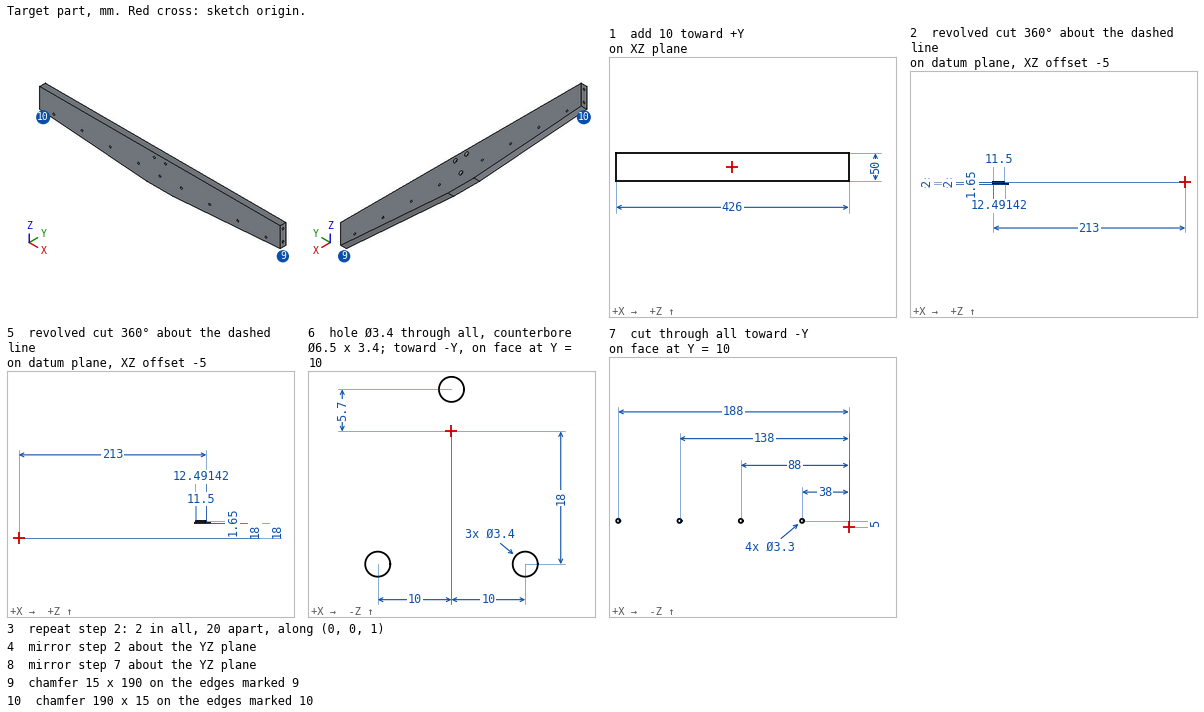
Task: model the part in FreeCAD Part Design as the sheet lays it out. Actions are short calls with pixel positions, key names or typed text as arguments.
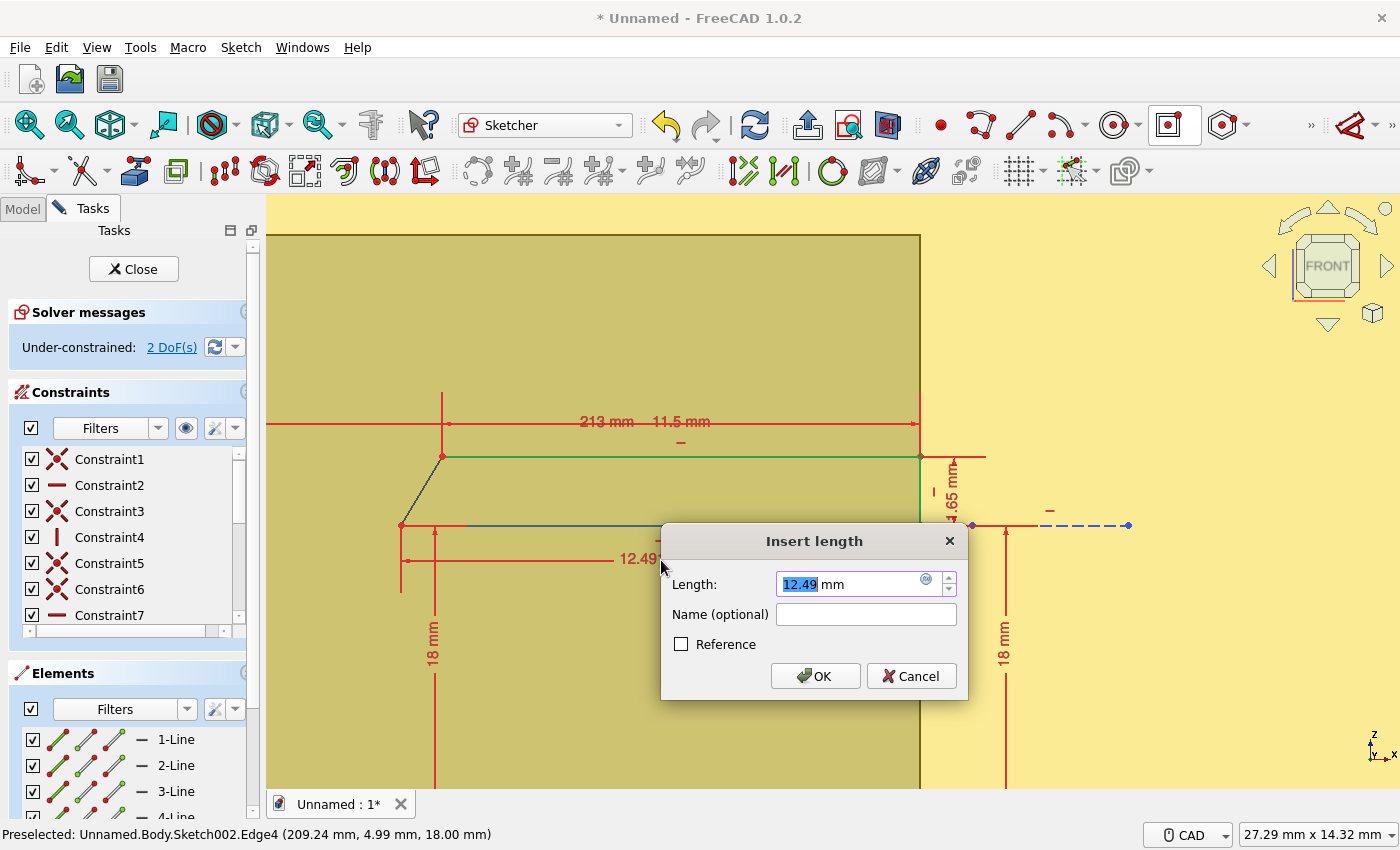
text(12.49142)
key(Return)
key(Escape)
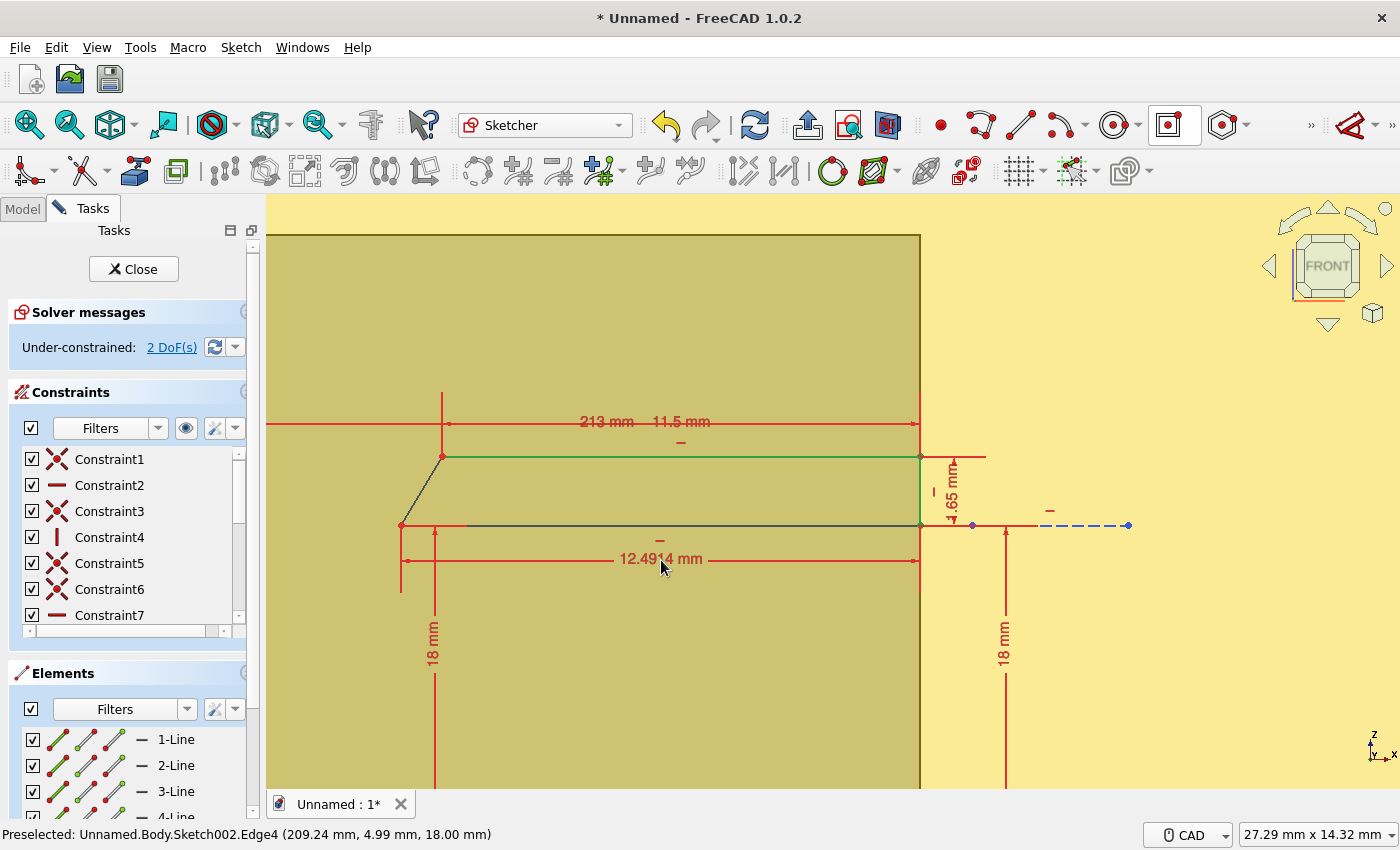
click(134, 269)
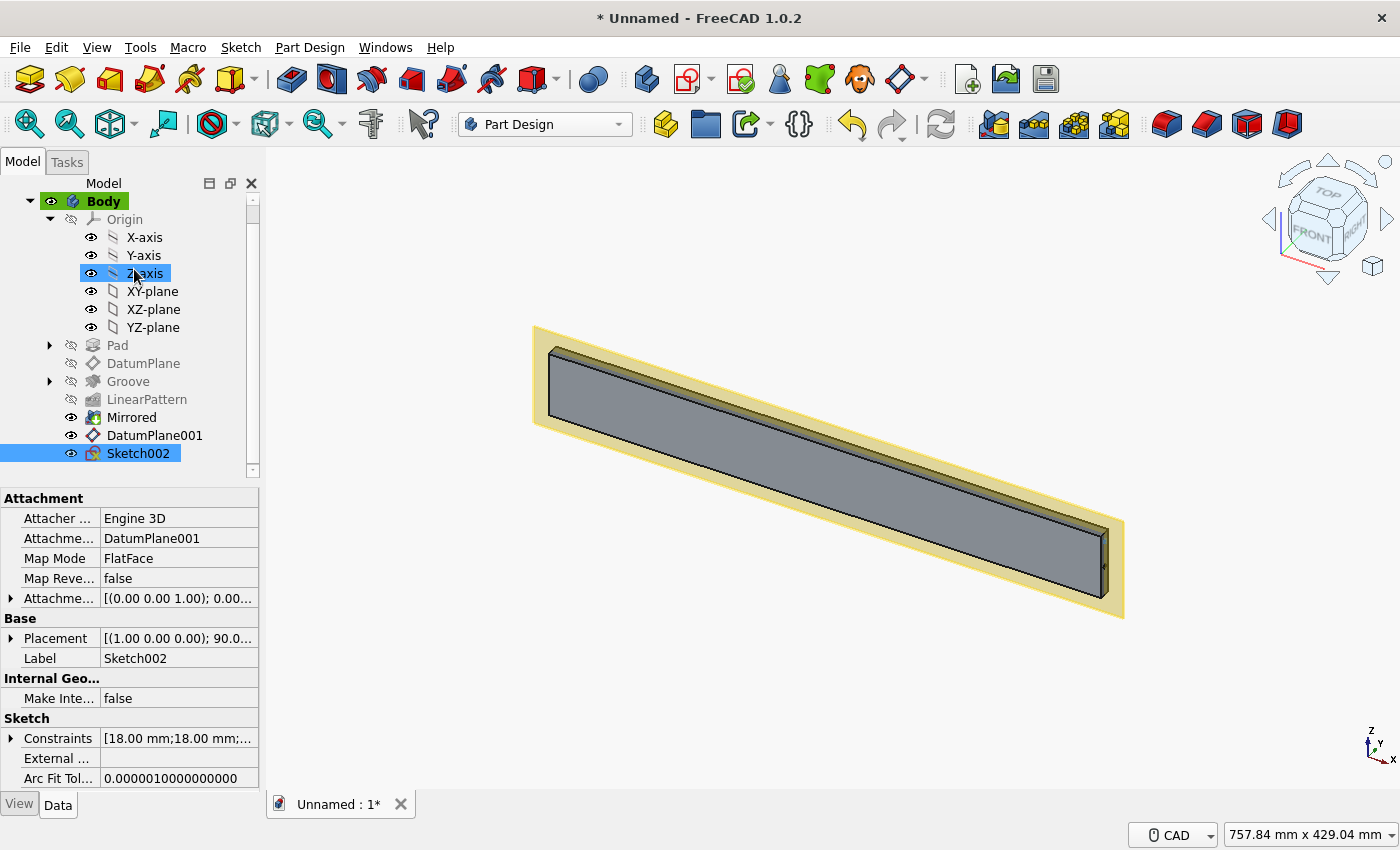
click(372, 80)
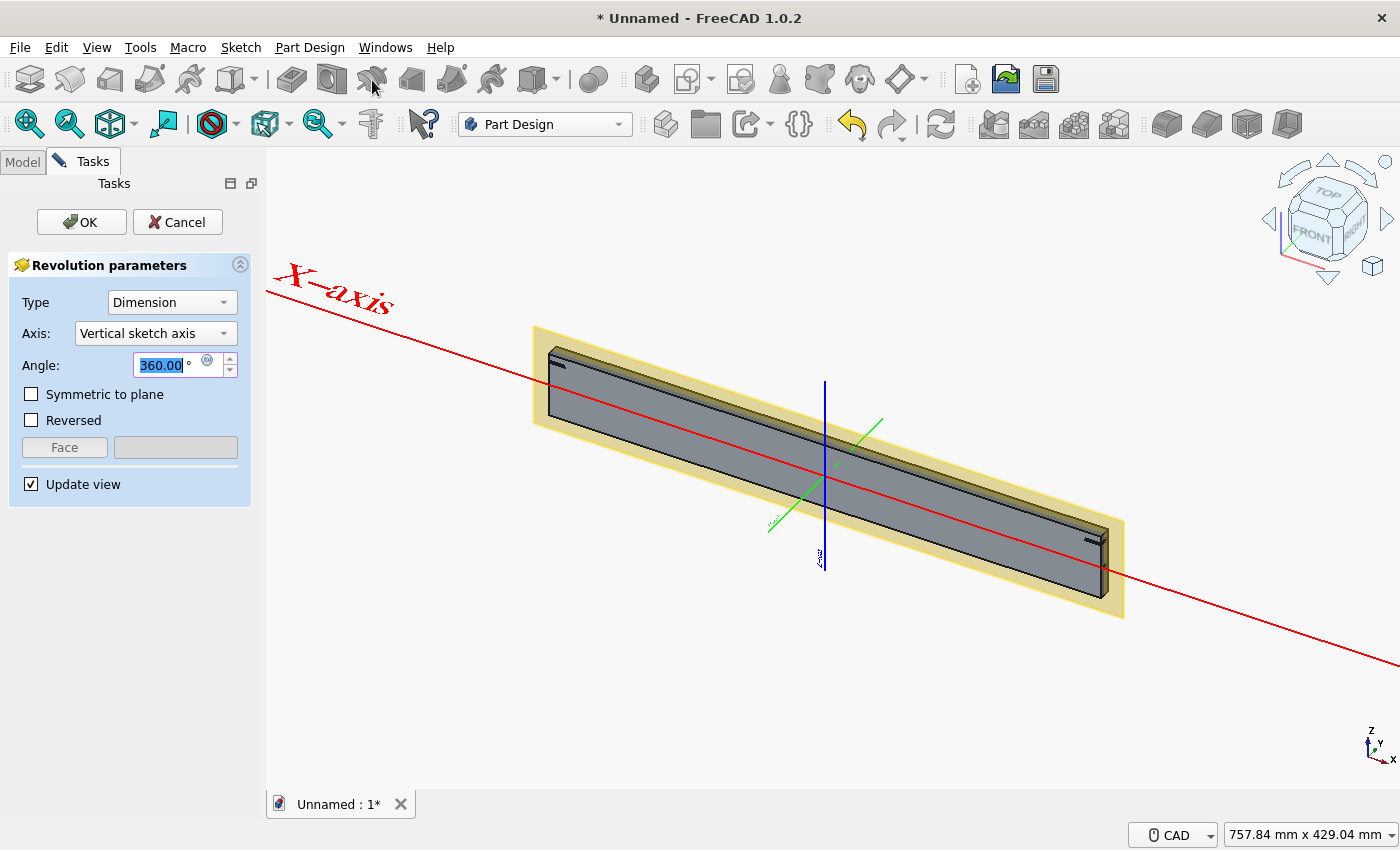
click(156, 334)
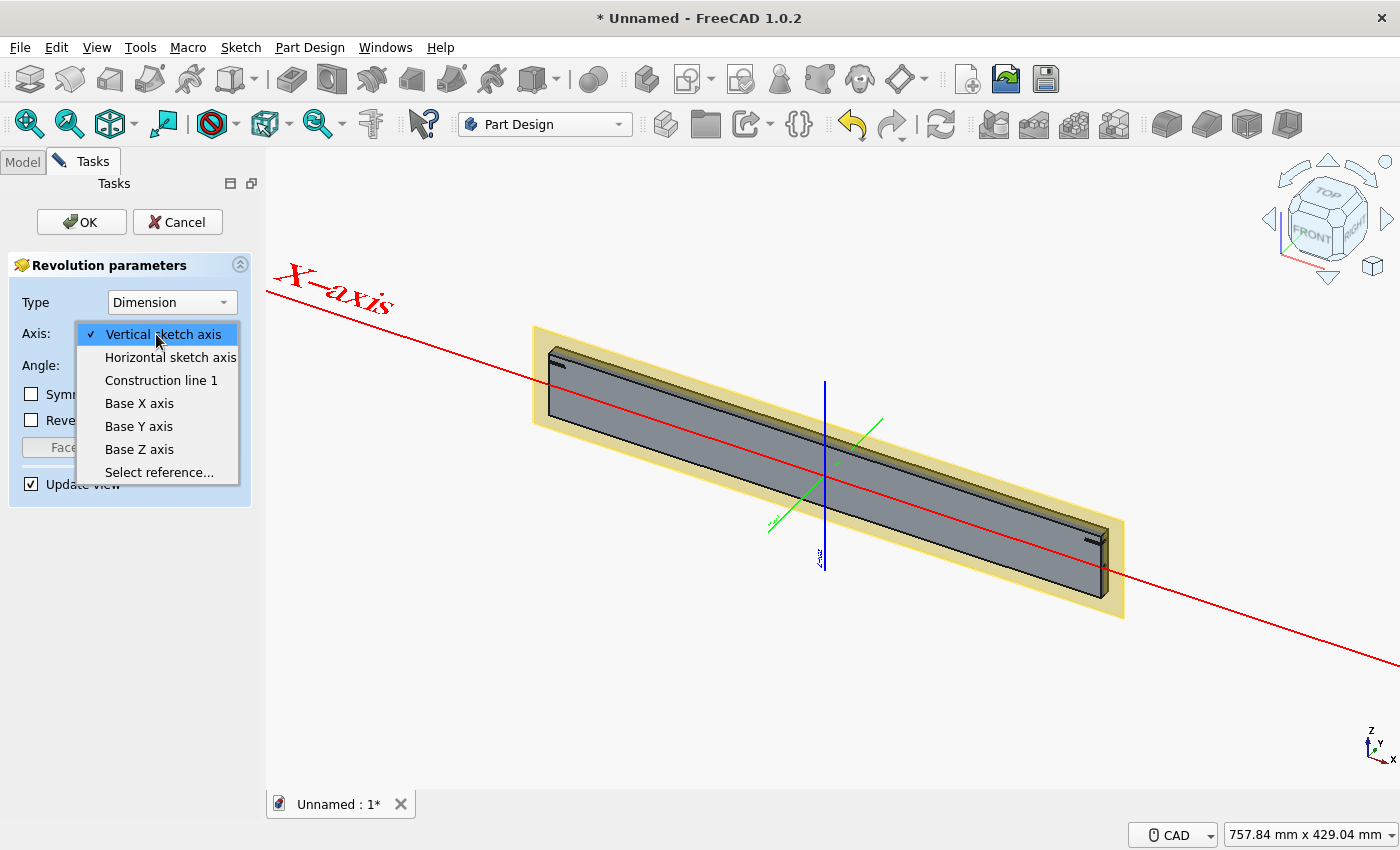
click(156, 380)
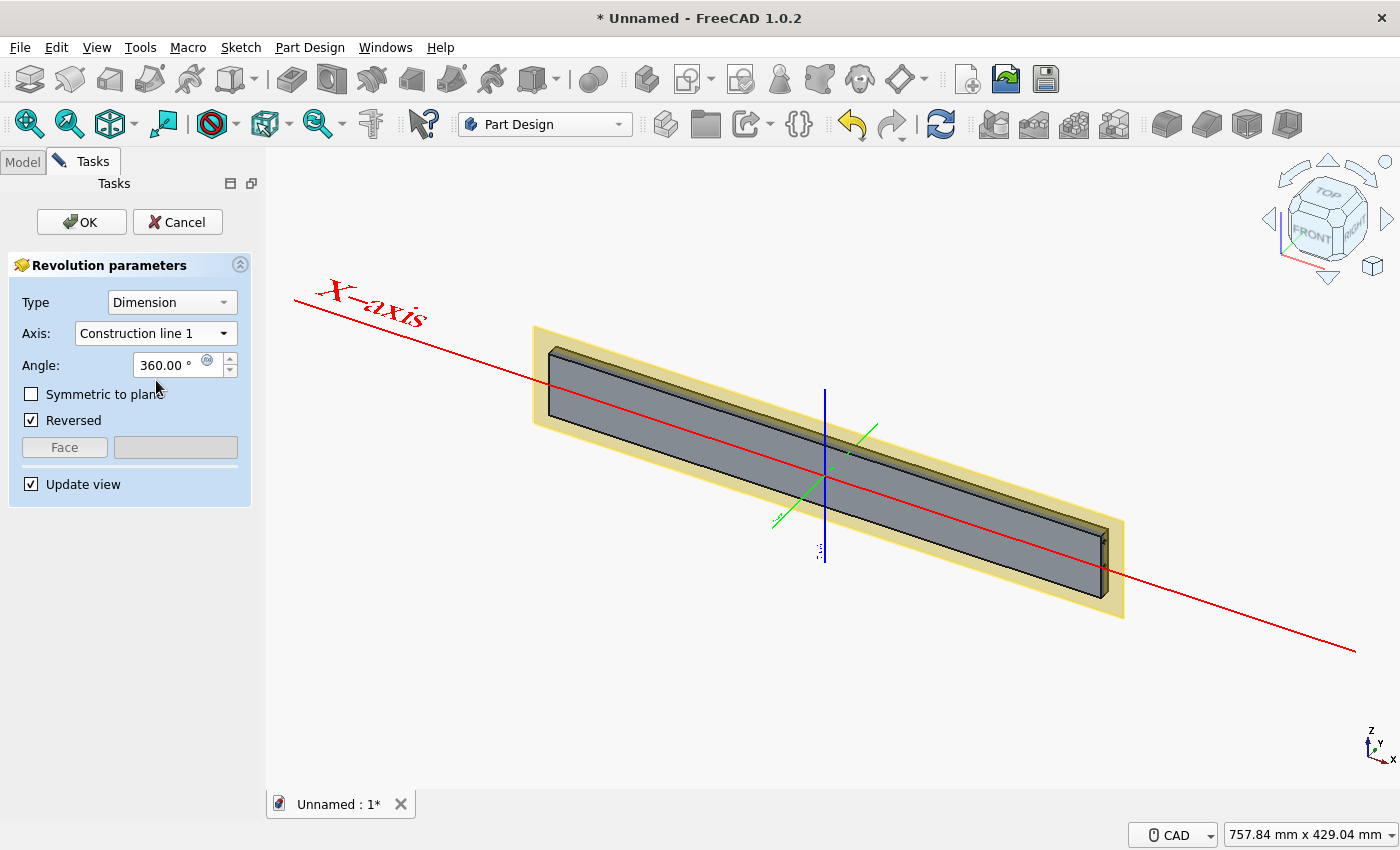
click(82, 222)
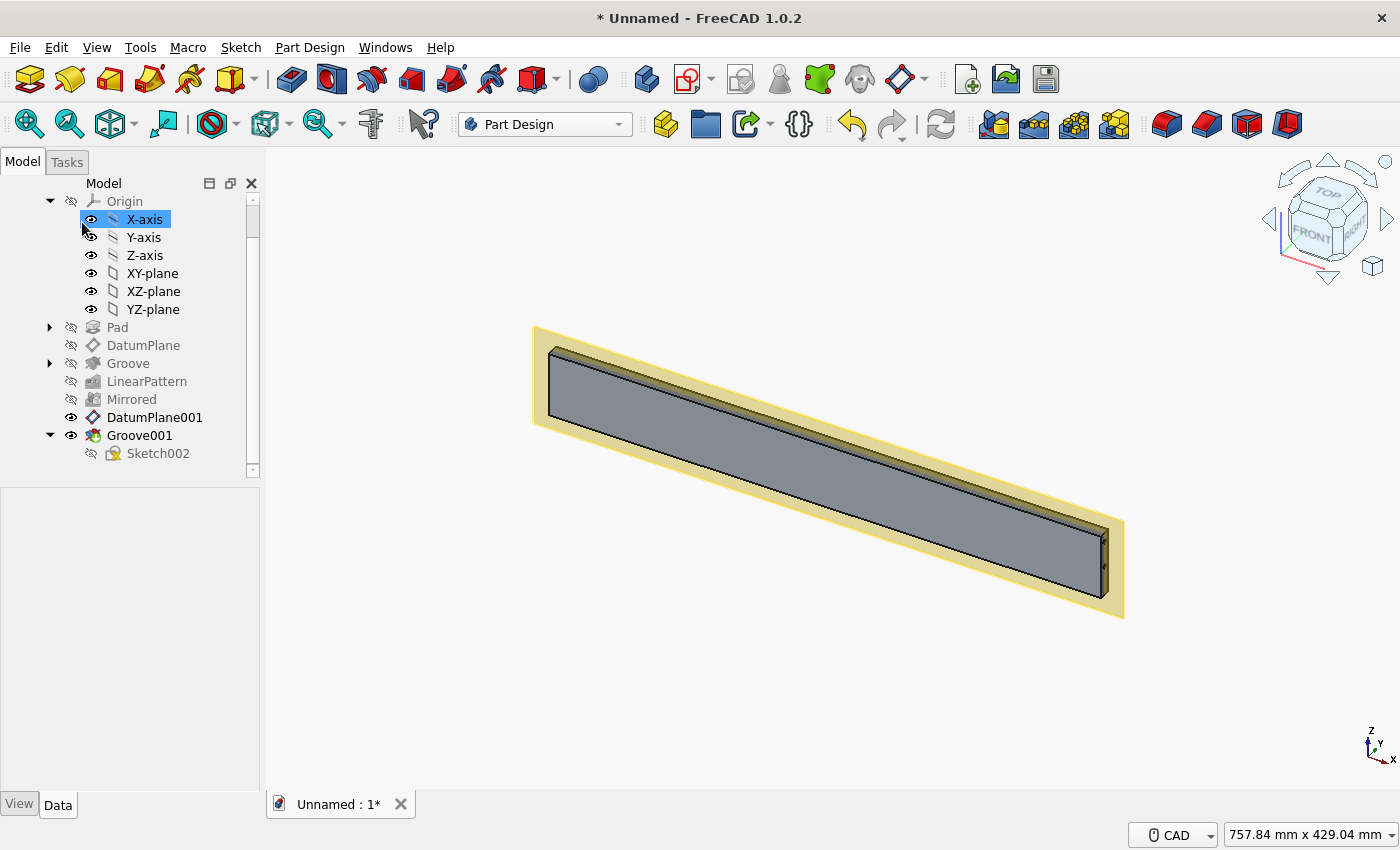
click(116, 417)
key(space)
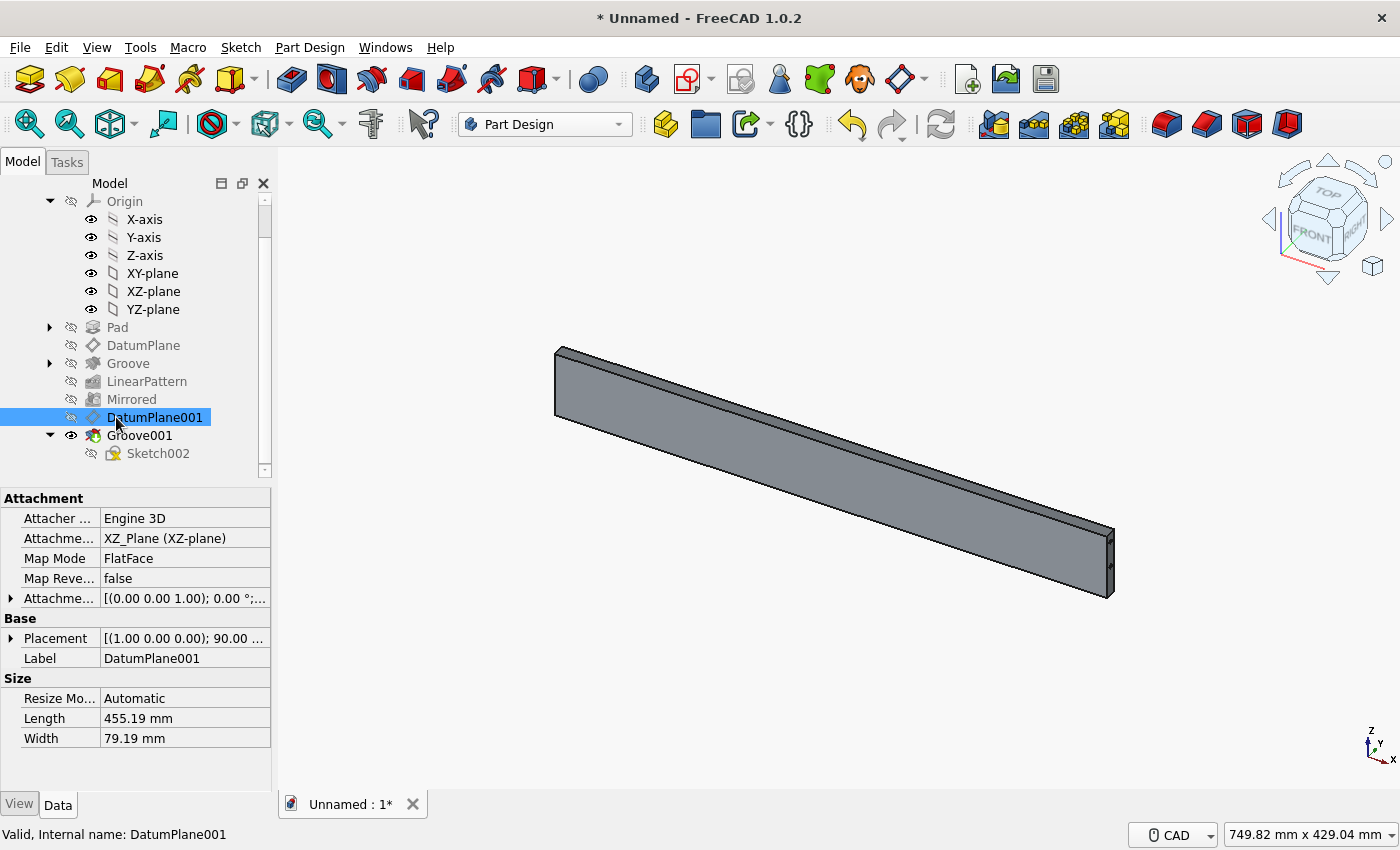
key(4)